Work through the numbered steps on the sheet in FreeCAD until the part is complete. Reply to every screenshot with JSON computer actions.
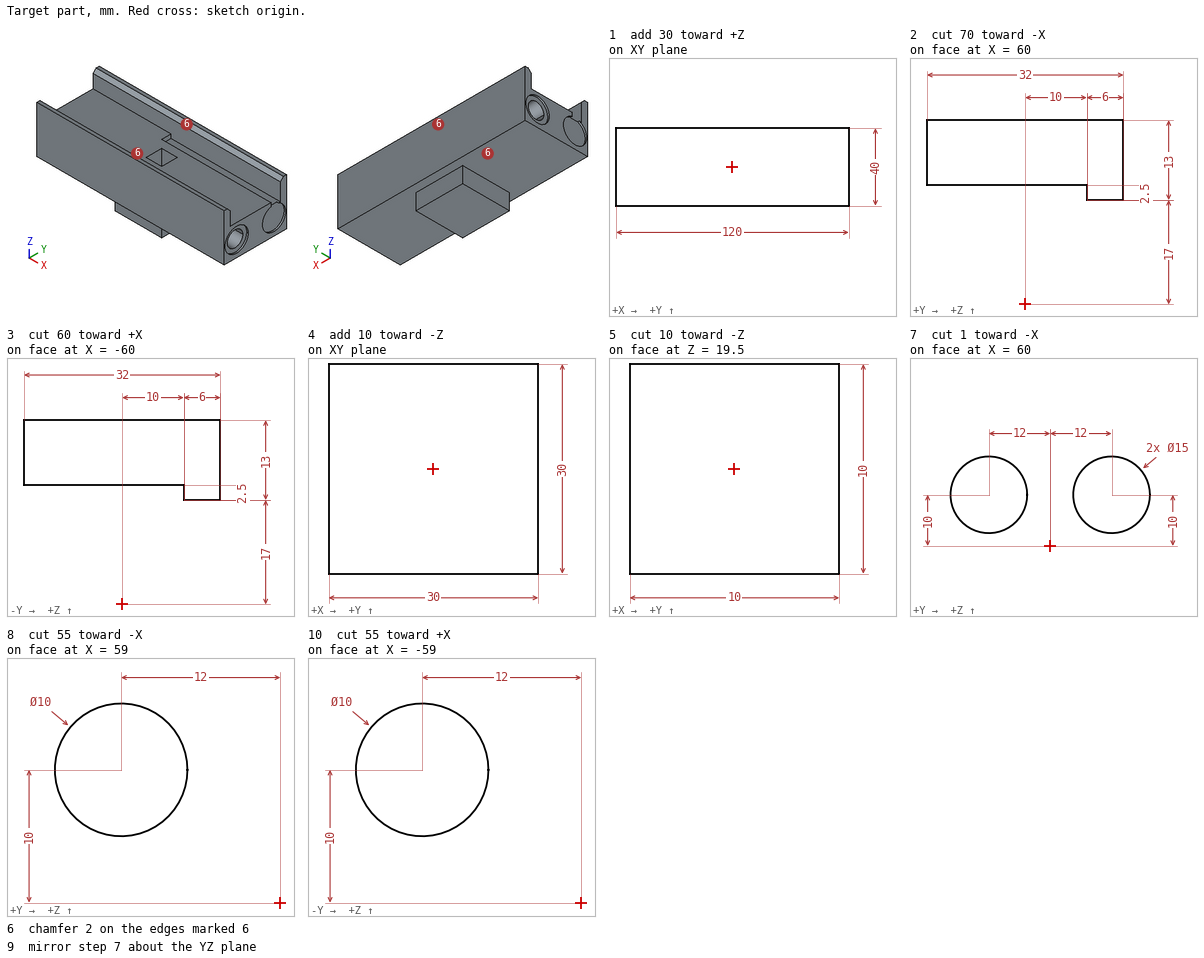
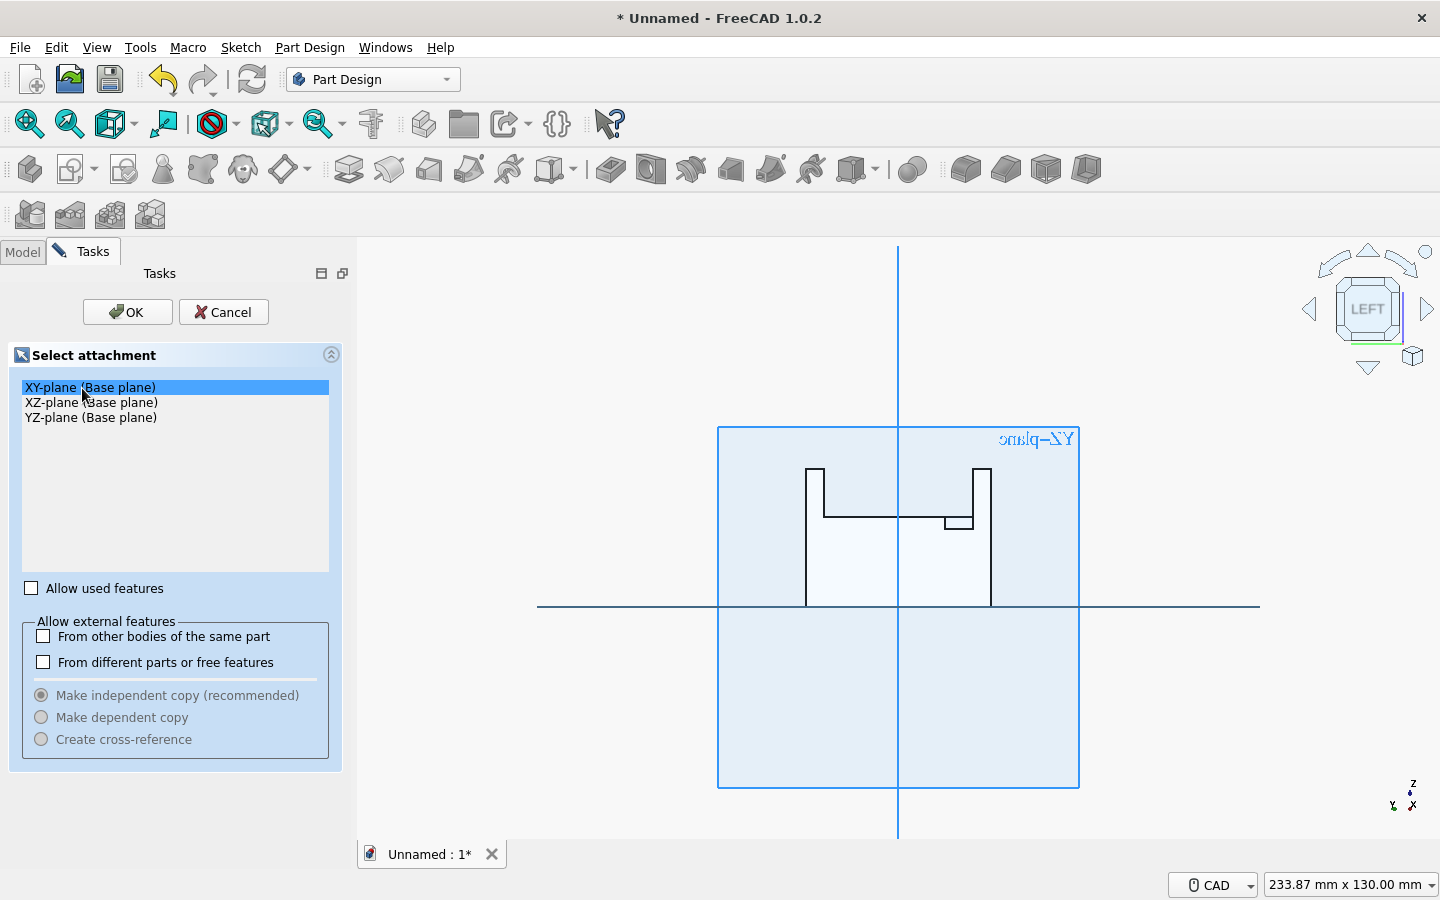
{"action": "left_click", "coordinate": [128, 312]}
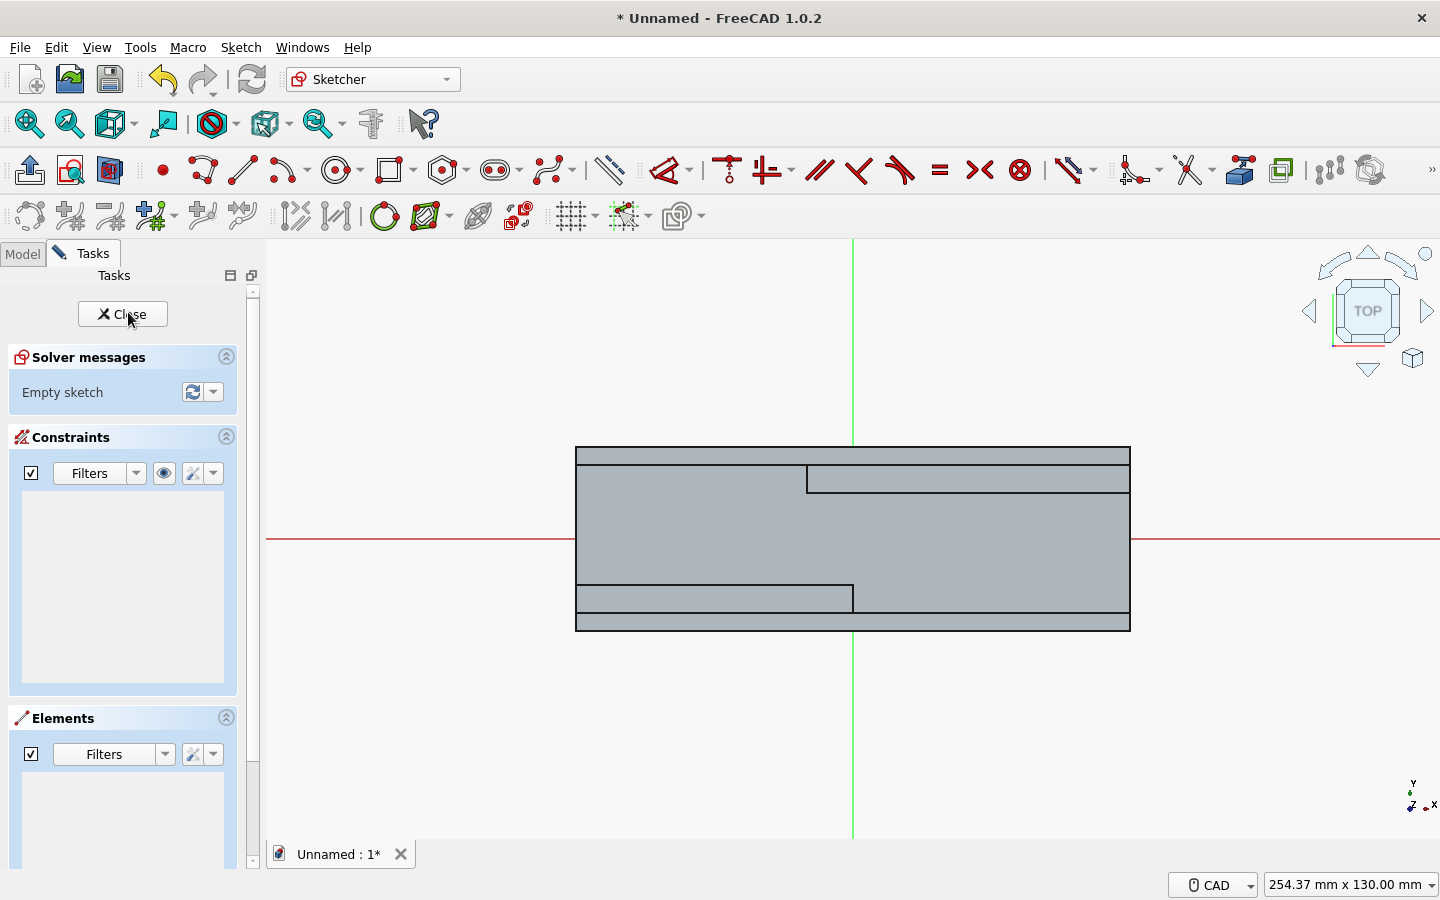
{"action": "key", "text": "q s"}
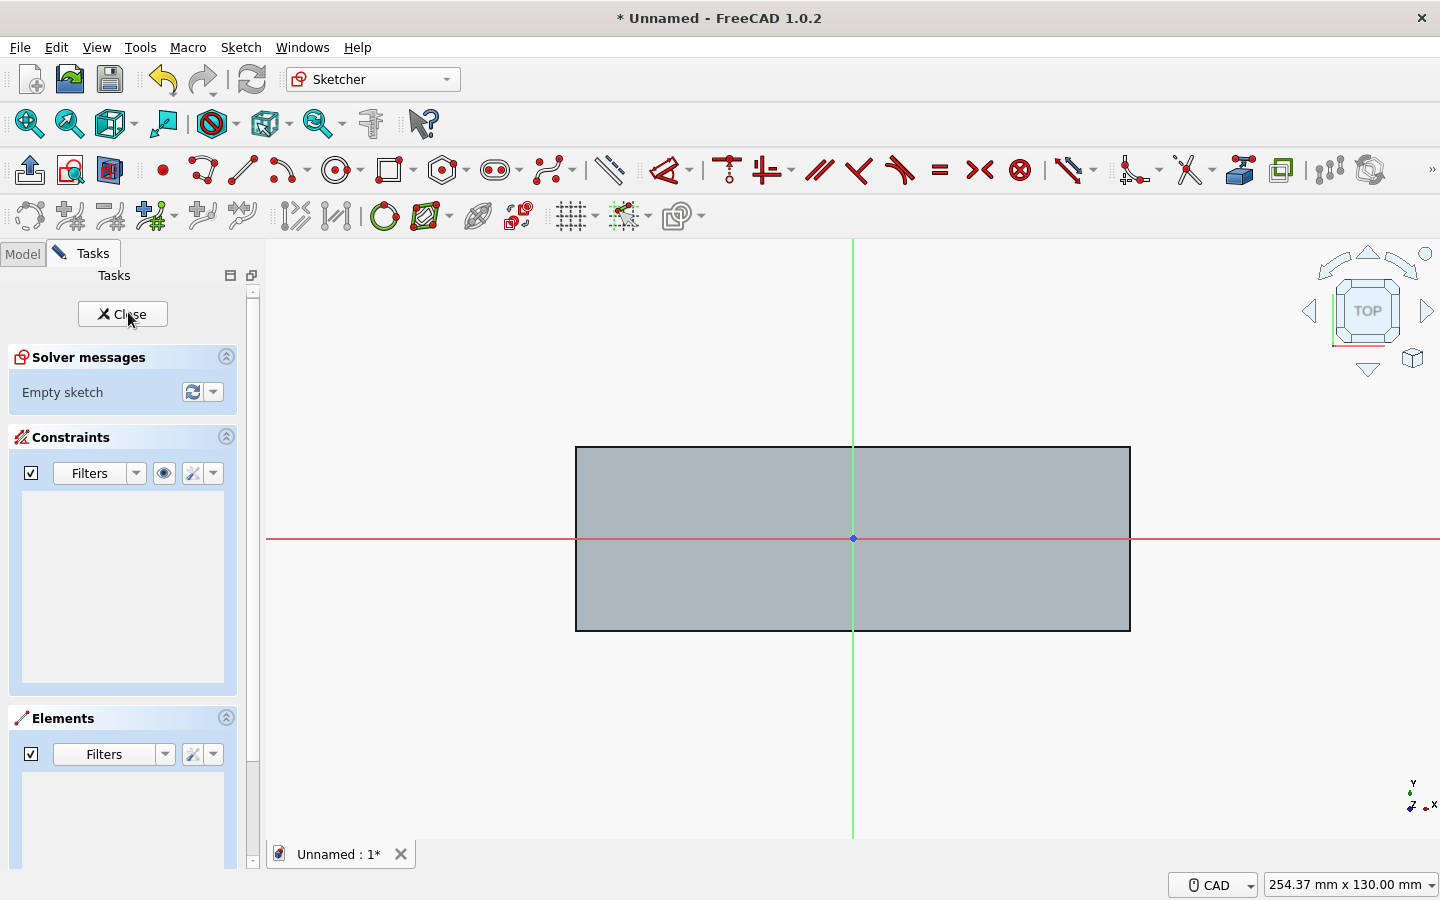
{"action": "scroll", "coordinate": [893, 539], "scroll_direction": "up", "scroll_amount": 5}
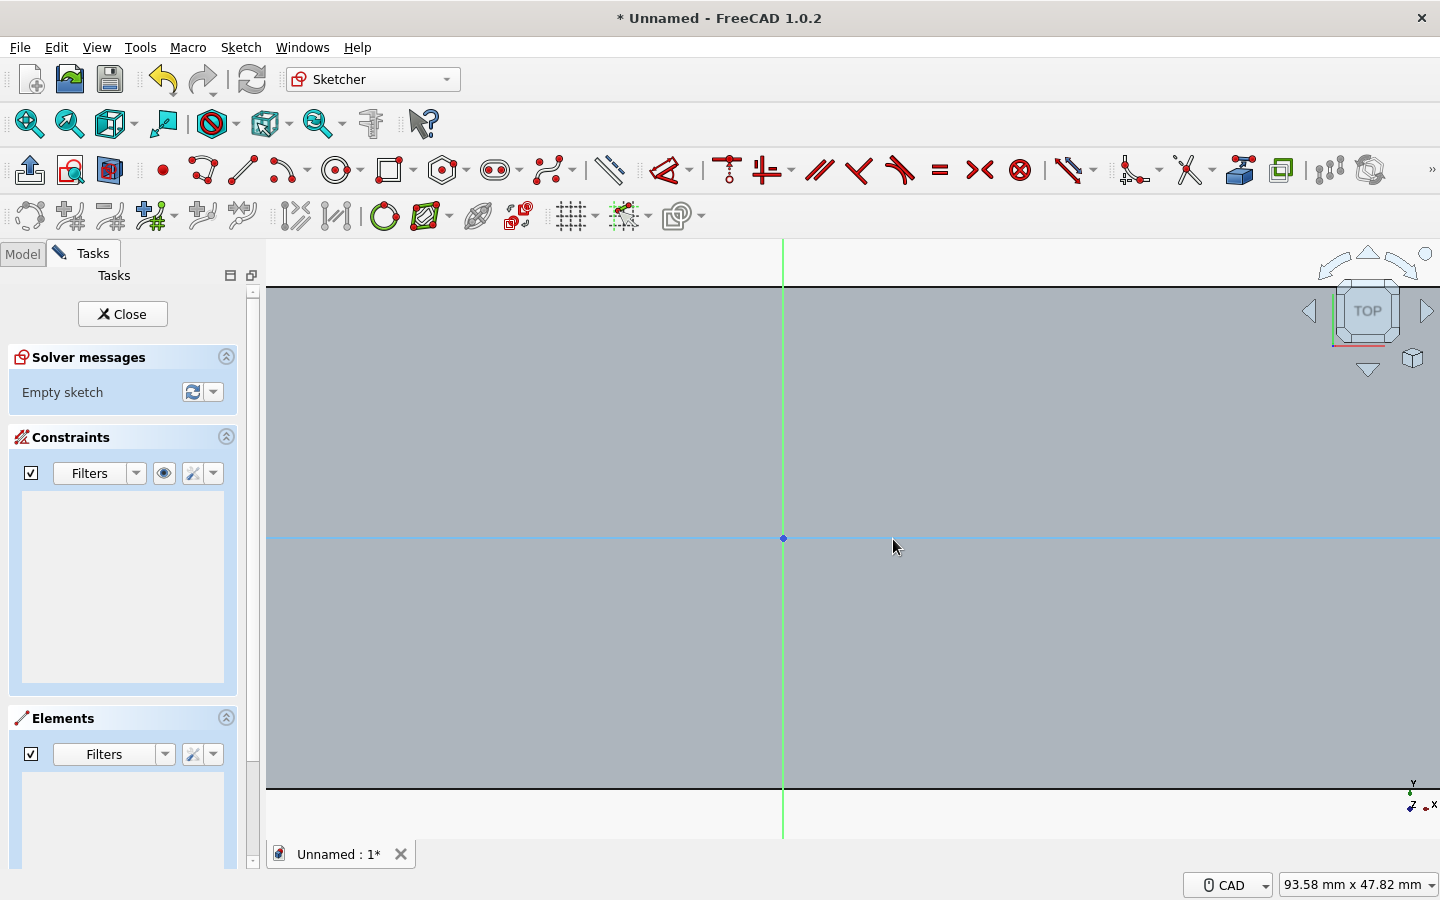
{"action": "key", "text": "g v"}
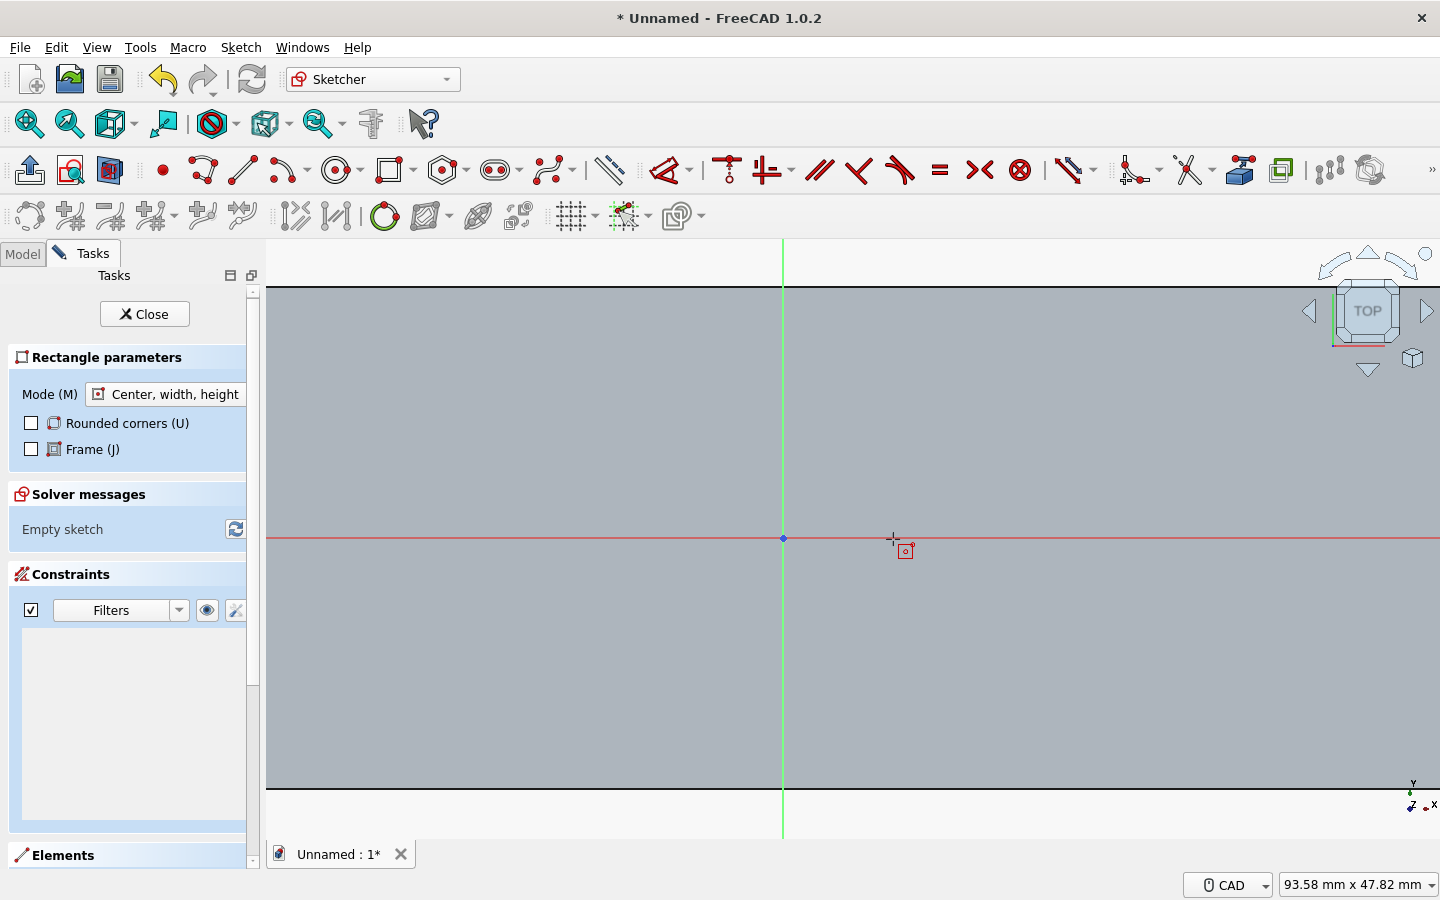
{"action": "left_click", "coordinate": [783, 538]}
{"action": "mouse_move", "coordinate": [972, 350]}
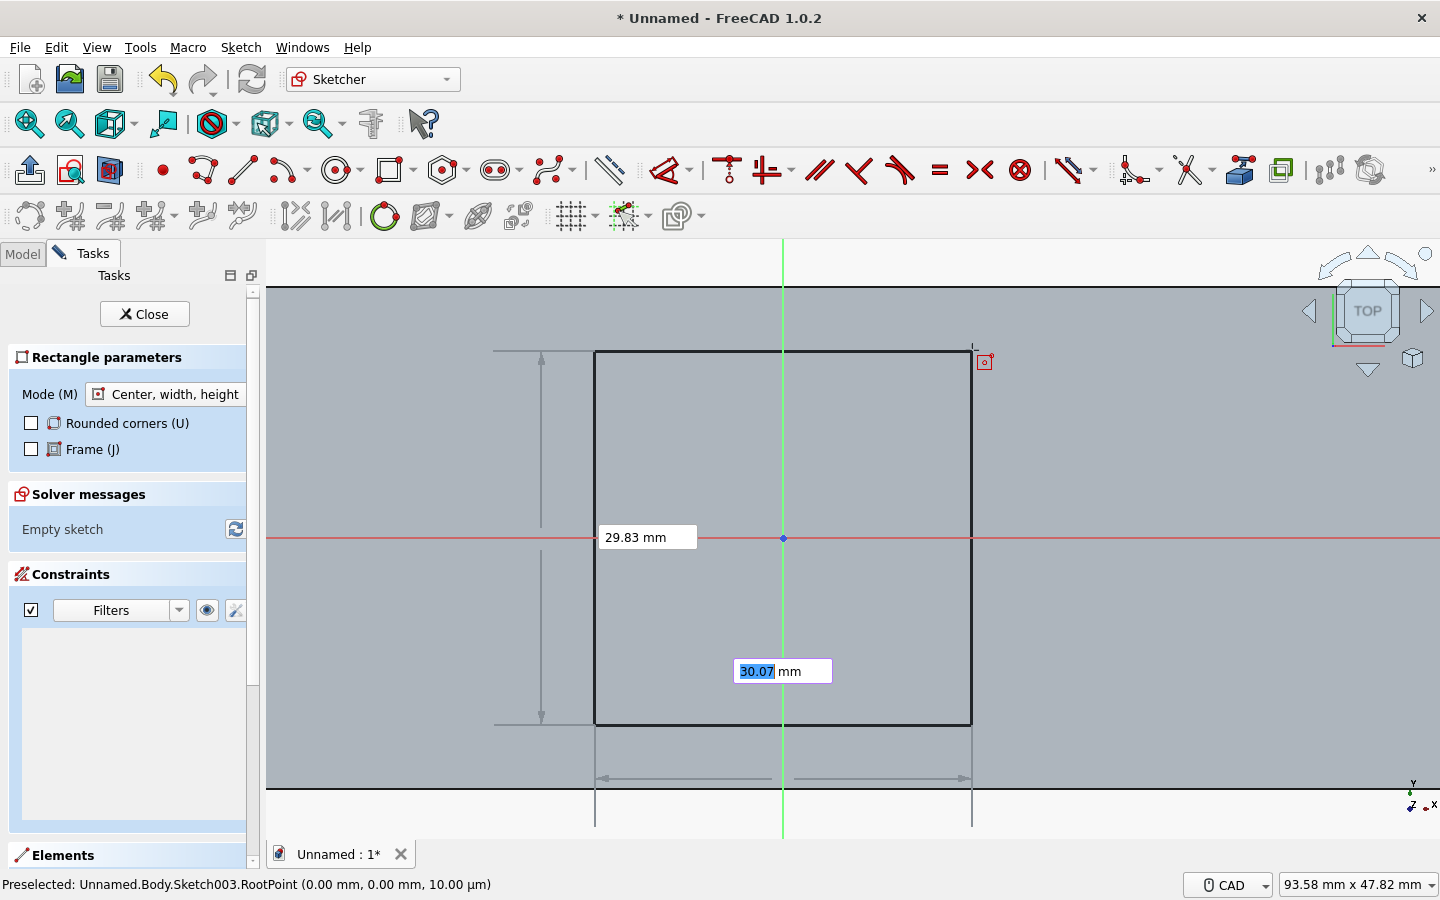
{"action": "type", "text": "30"}
{"action": "key", "text": "Tab"}
{"action": "type", "text": "30"}
{"action": "key", "text": "Return"}
{"action": "key", "text": "Escape"}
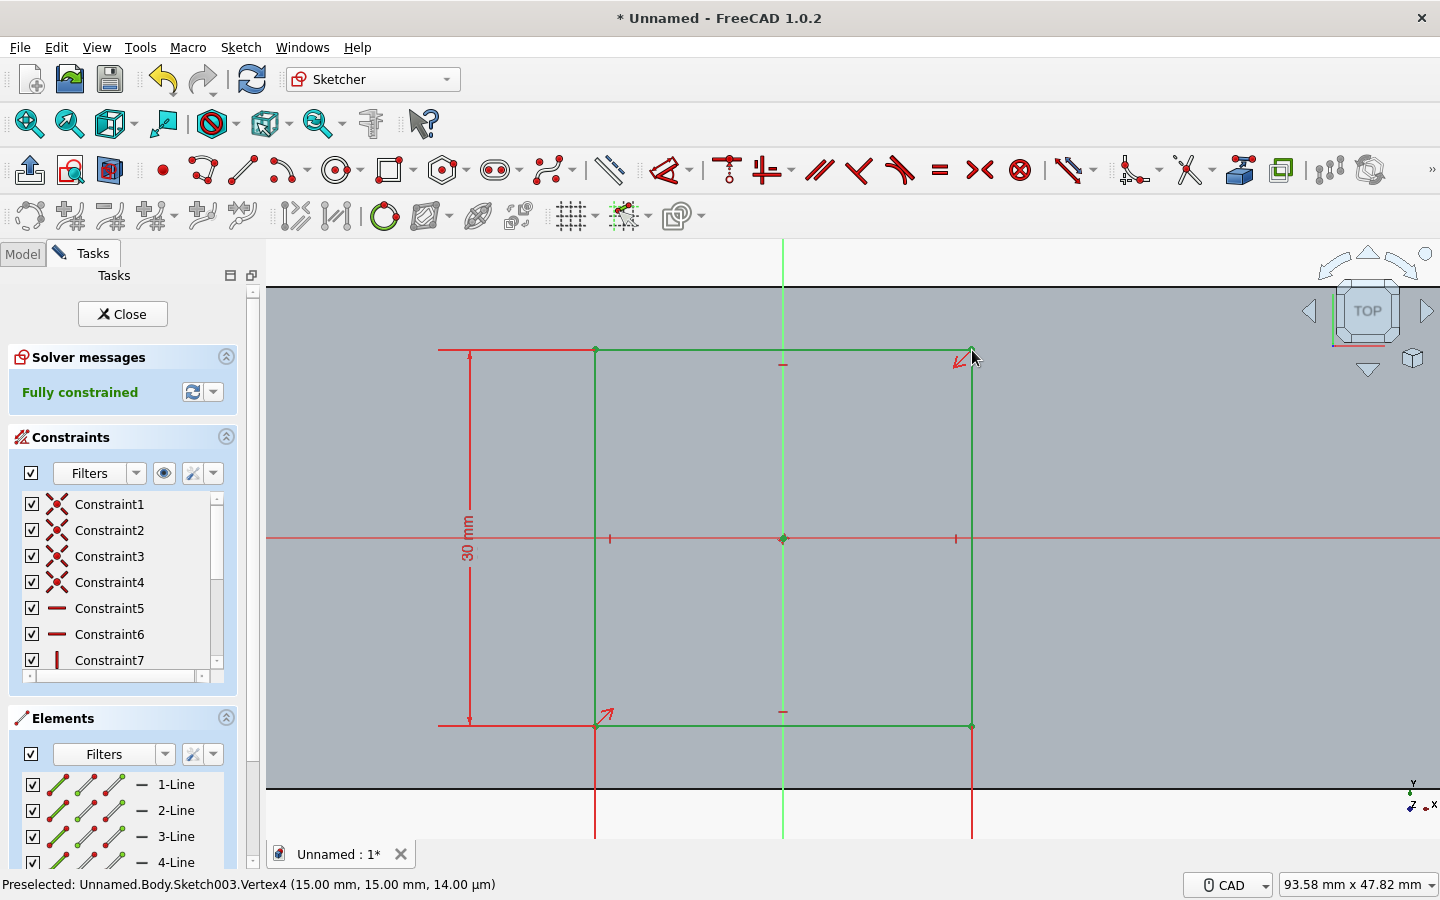
{"action": "left_click", "coordinate": [123, 314]}